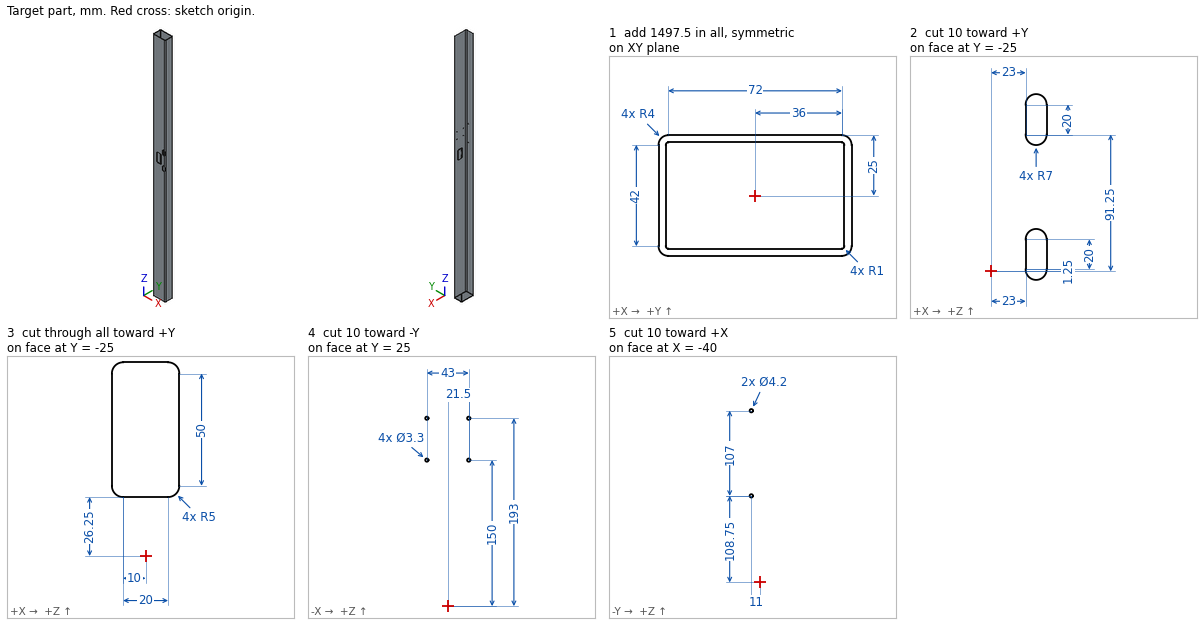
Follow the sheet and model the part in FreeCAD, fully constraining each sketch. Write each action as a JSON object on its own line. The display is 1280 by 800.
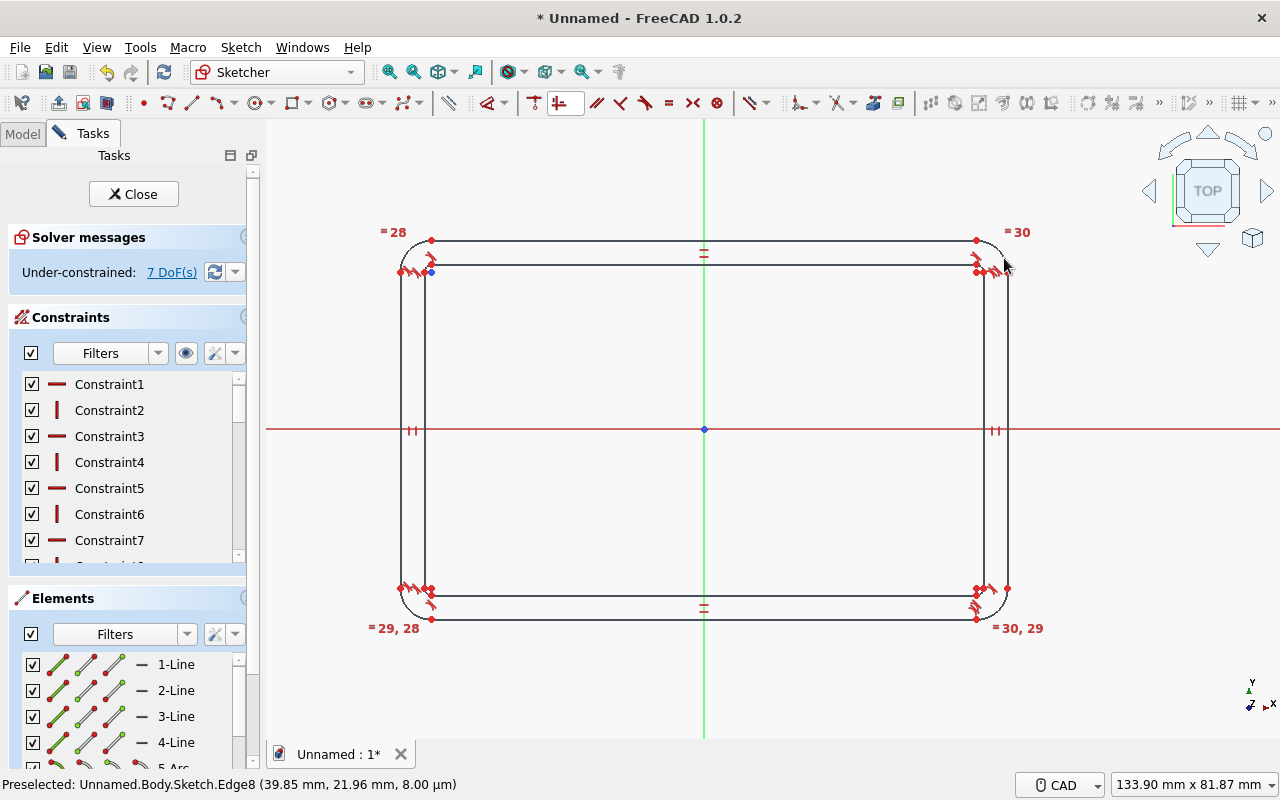
{"action": "scroll", "coordinate": [981, 267], "scroll_direction": "up", "scroll_amount": 5}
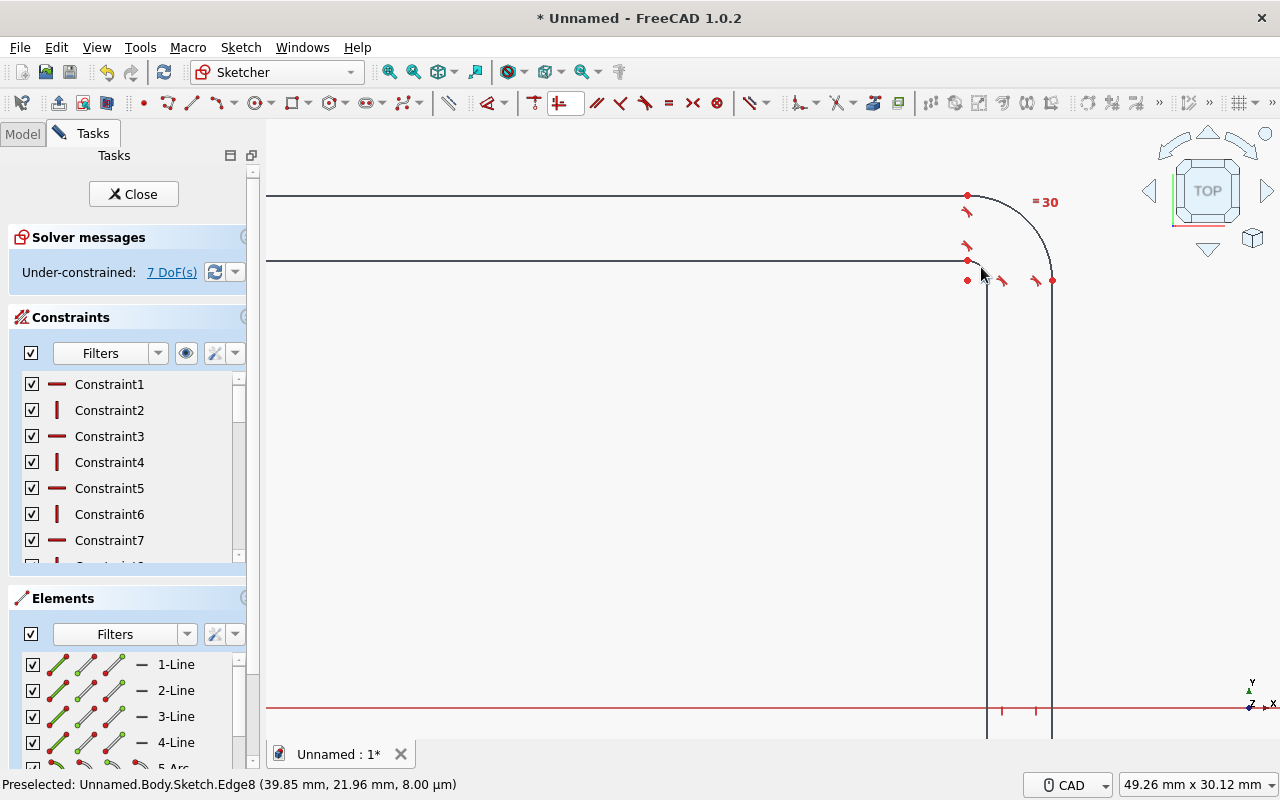
{"action": "left_click", "coordinate": [981, 267]}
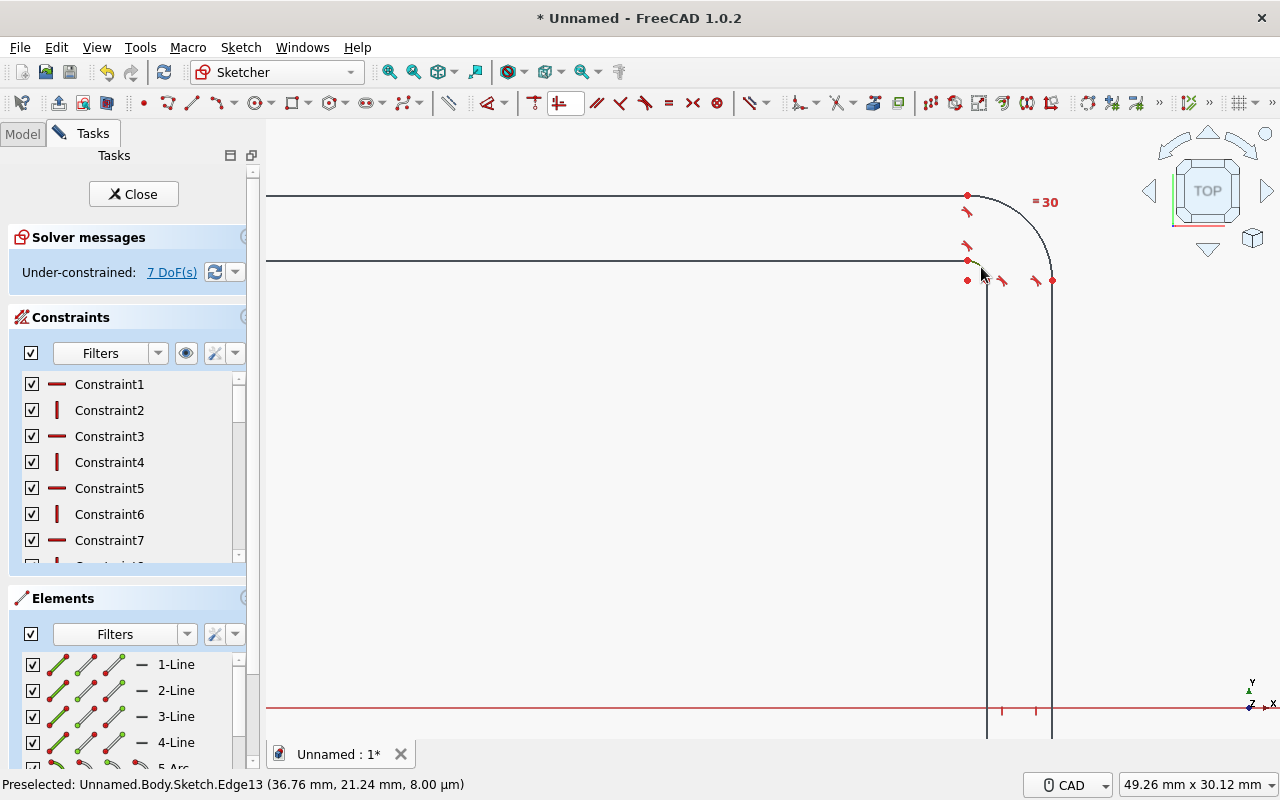
{"action": "scroll", "coordinate": [982, 266], "scroll_direction": "down", "scroll_amount": 5}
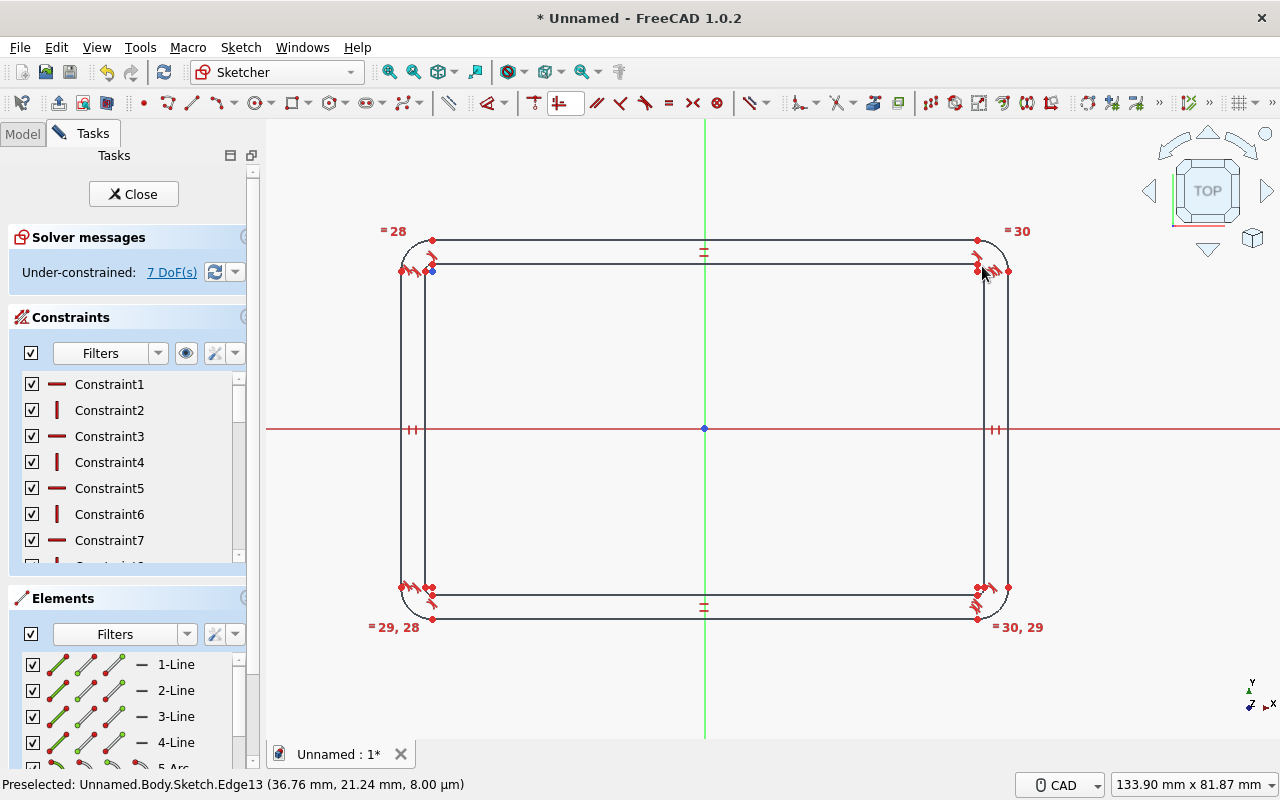
{"action": "scroll", "coordinate": [429, 265], "scroll_direction": "up", "scroll_amount": 7}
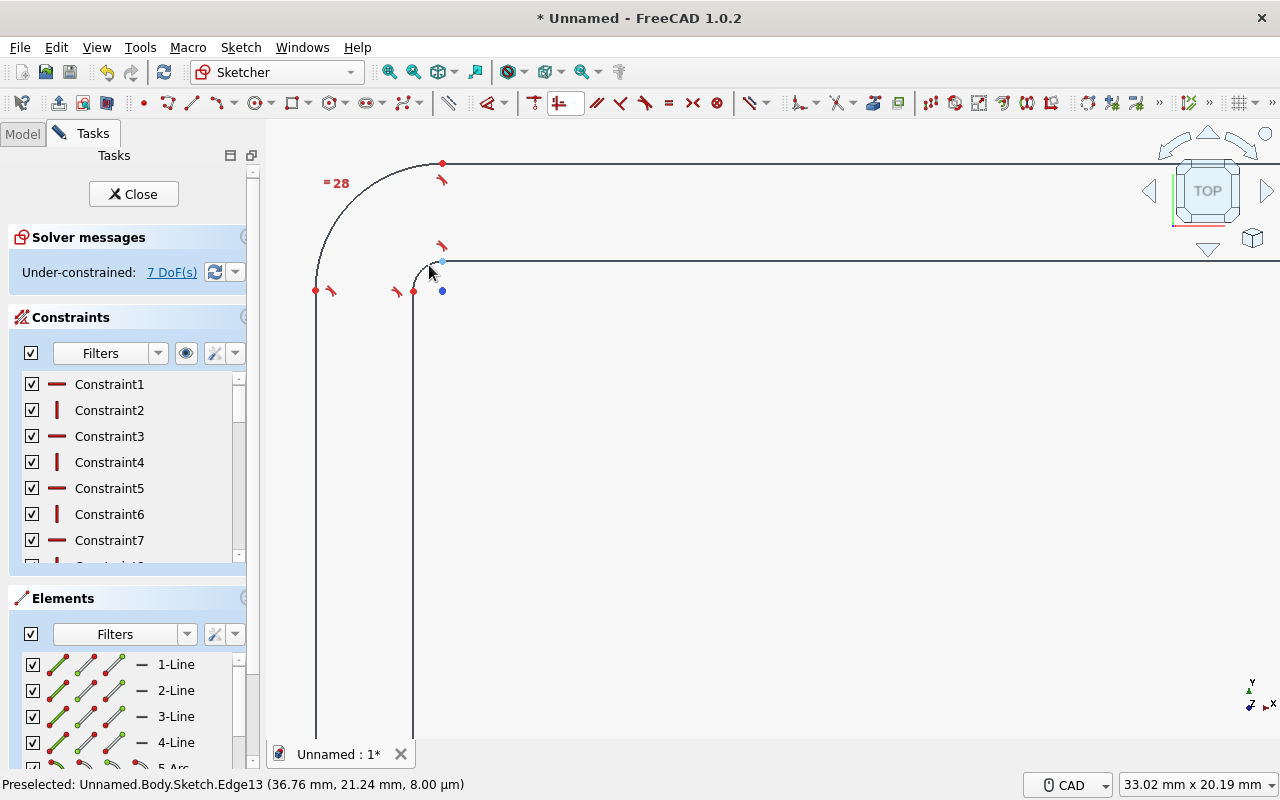
{"action": "left_click", "coordinate": [429, 265]}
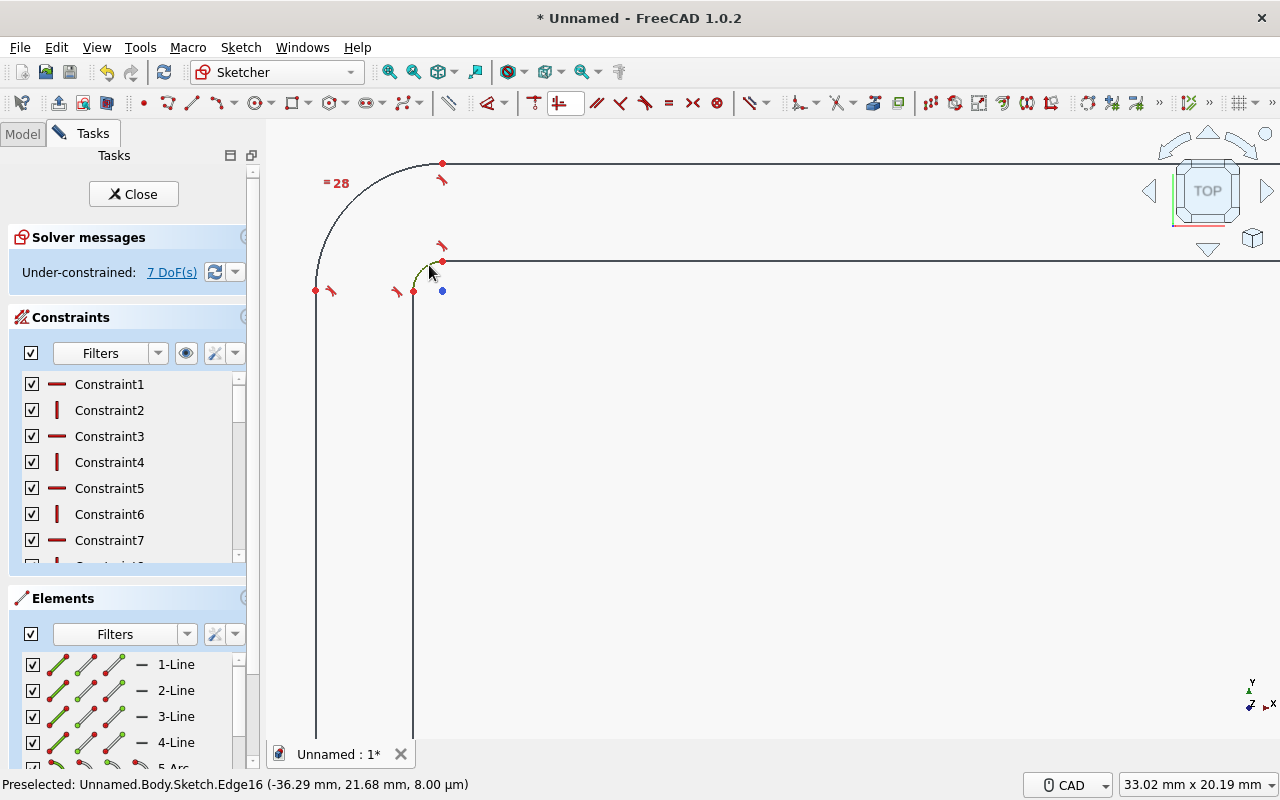
{"action": "key", "text": "e"}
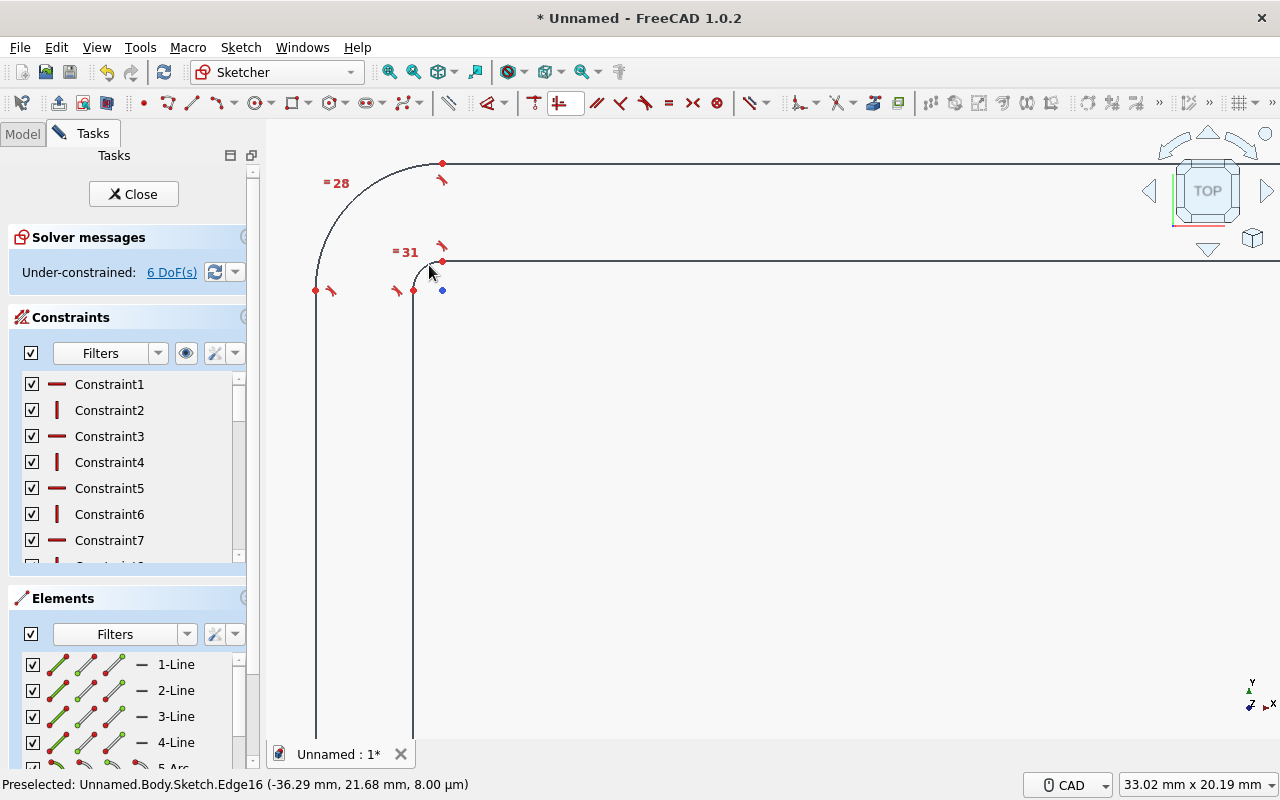
{"action": "key", "text": "d"}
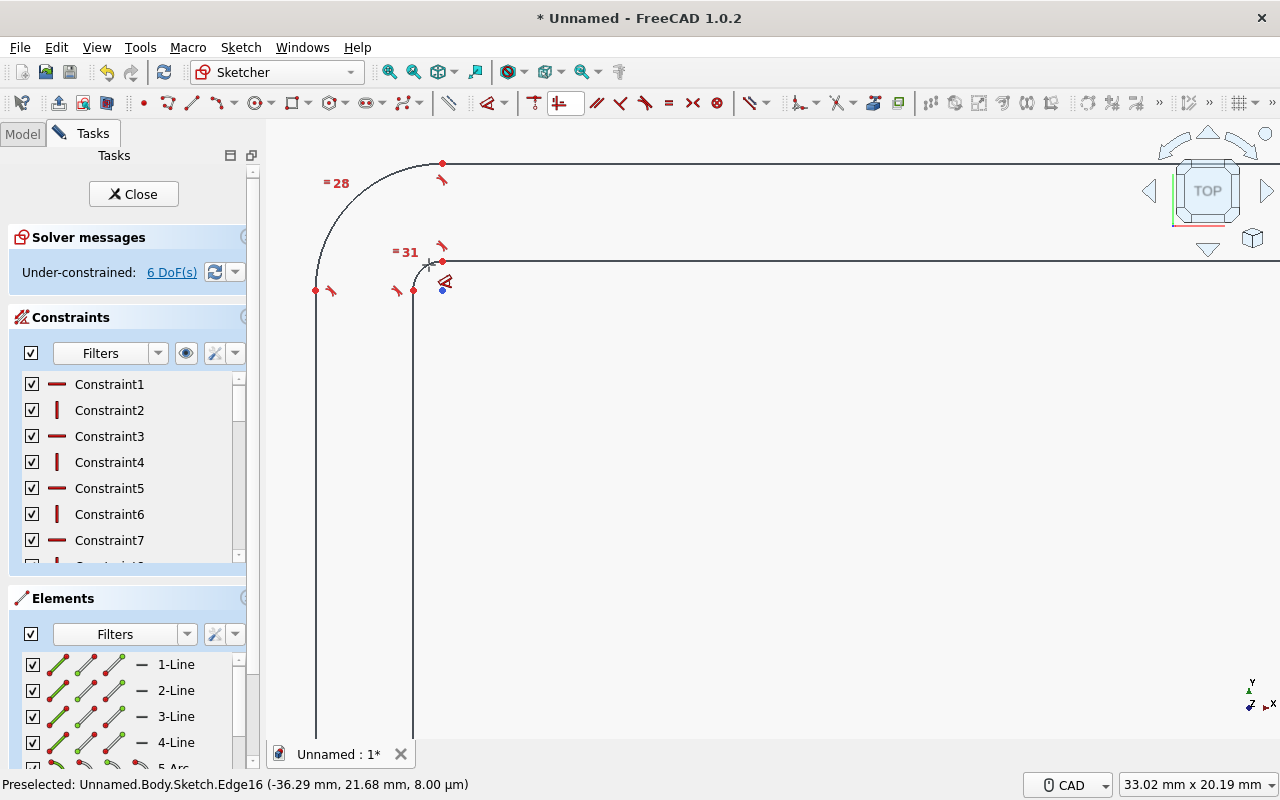
{"action": "scroll", "coordinate": [429, 265], "scroll_direction": "down", "scroll_amount": 7}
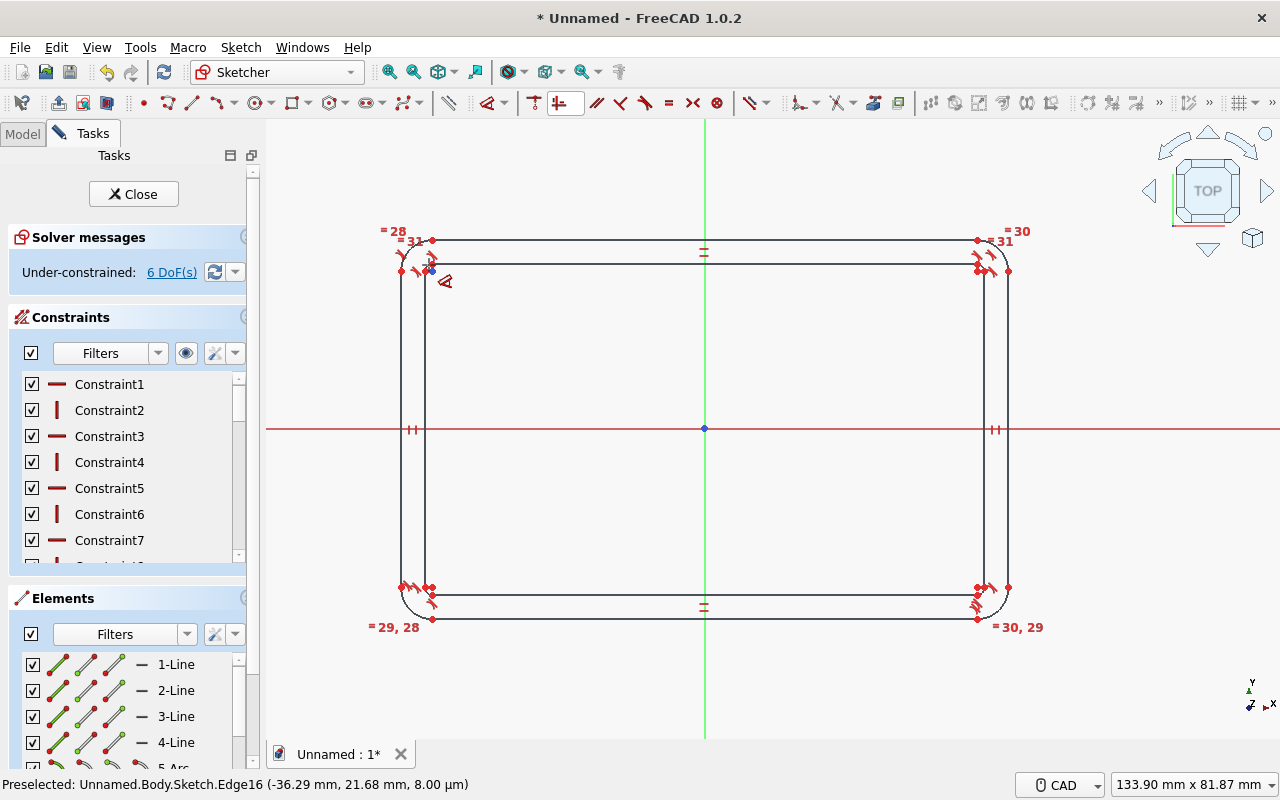
{"action": "scroll", "coordinate": [418, 244], "scroll_direction": "up", "scroll_amount": 2}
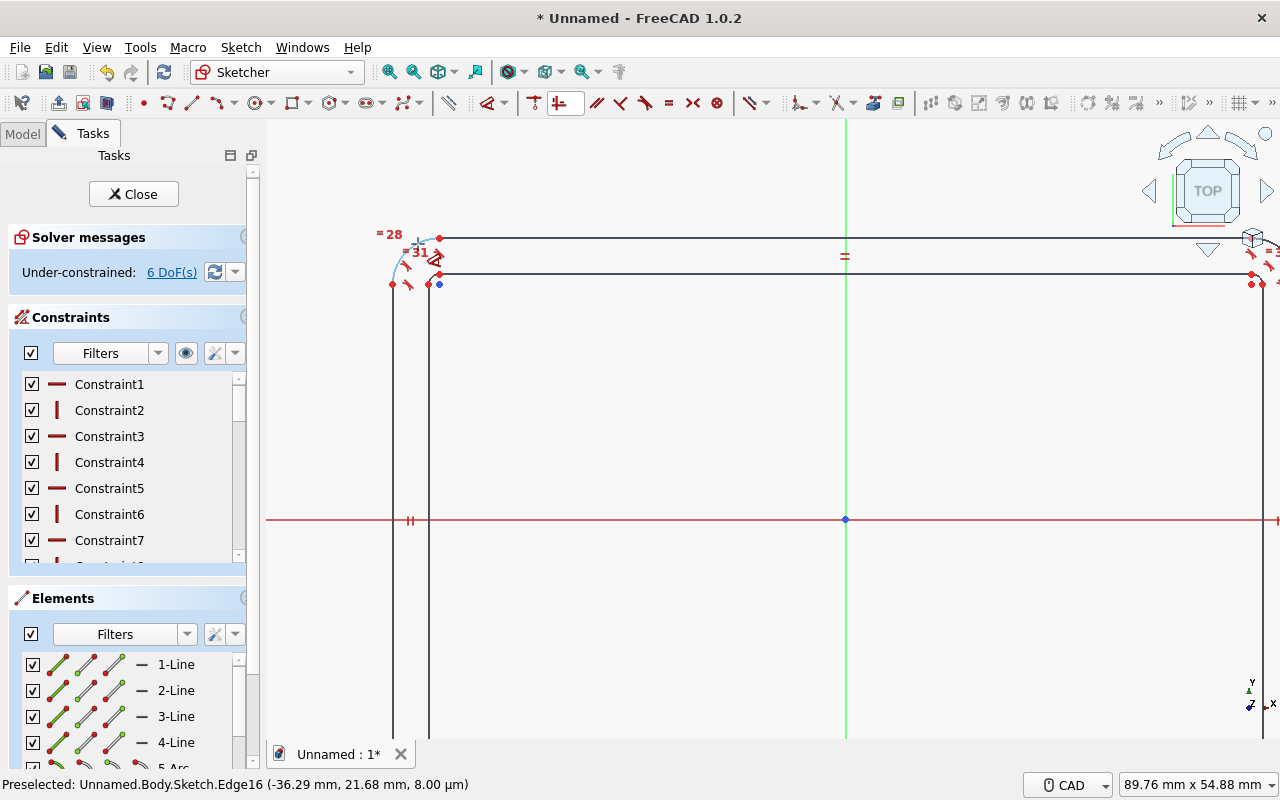
{"action": "left_click", "coordinate": [418, 243]}
{"action": "left_click", "coordinate": [403, 214]}